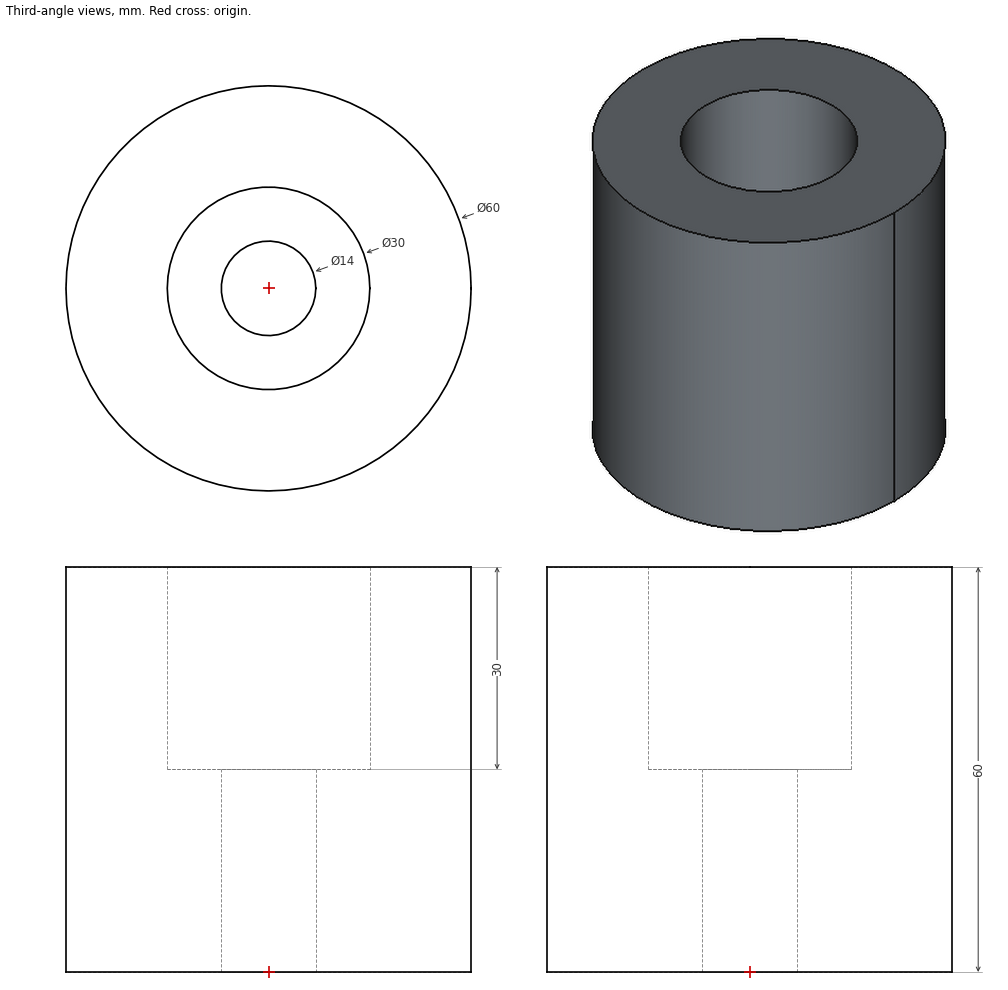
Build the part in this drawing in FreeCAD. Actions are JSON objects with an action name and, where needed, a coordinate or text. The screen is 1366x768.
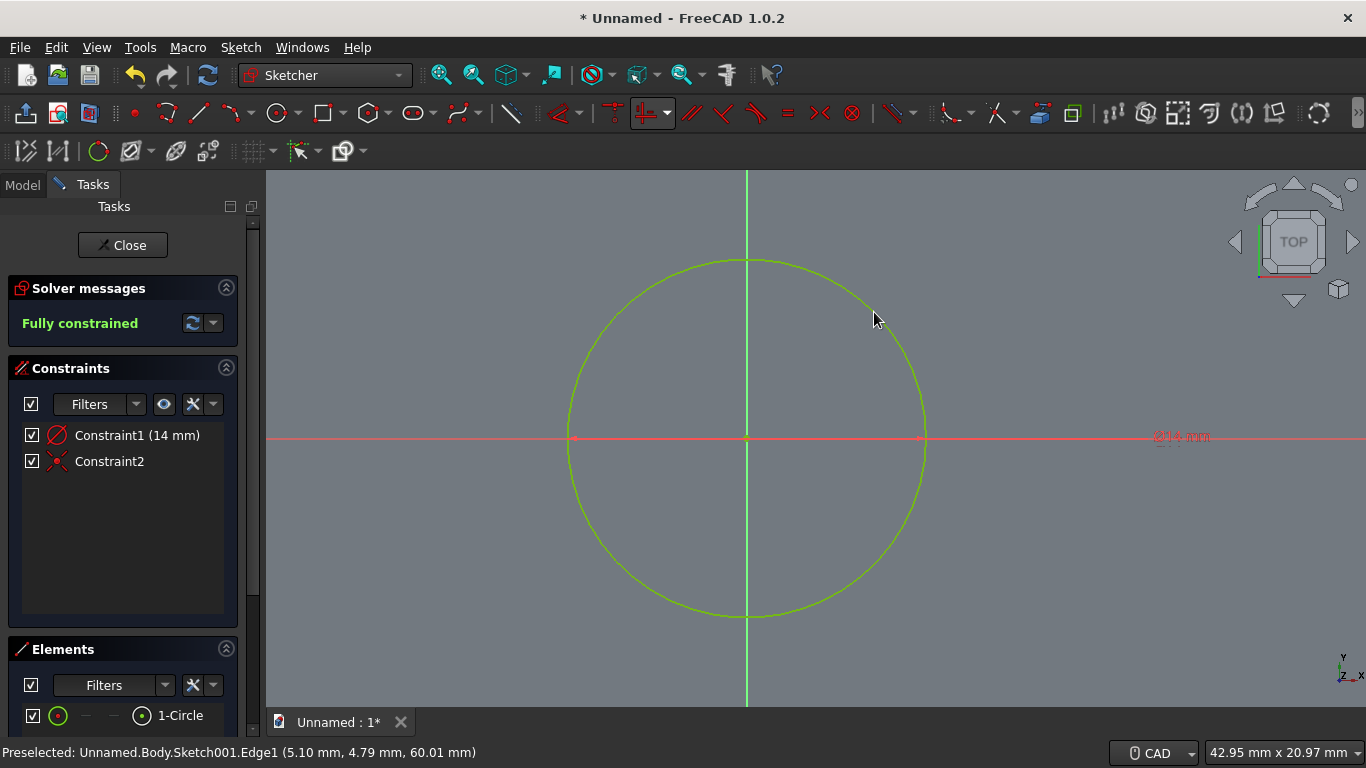
{"action": "left_click", "coordinate": [123, 245]}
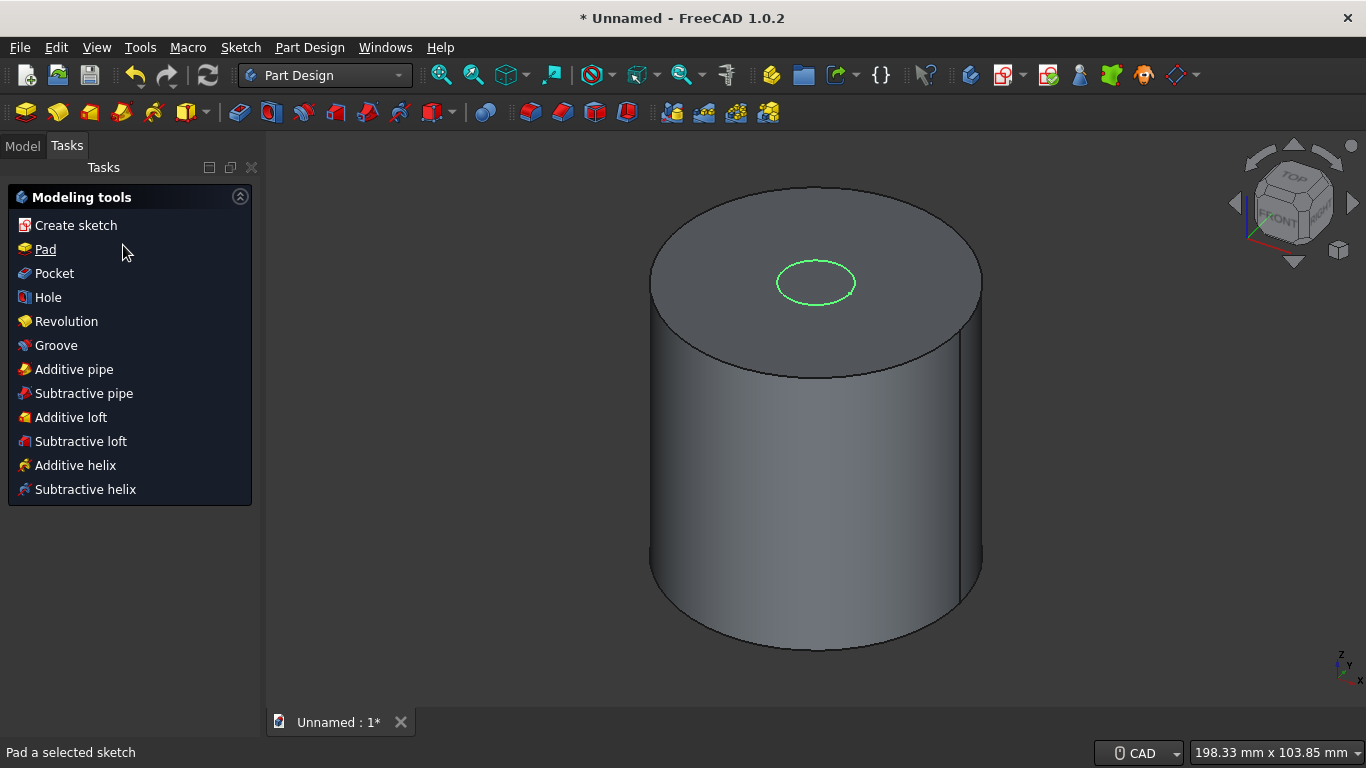
{"action": "left_click", "coordinate": [240, 112]}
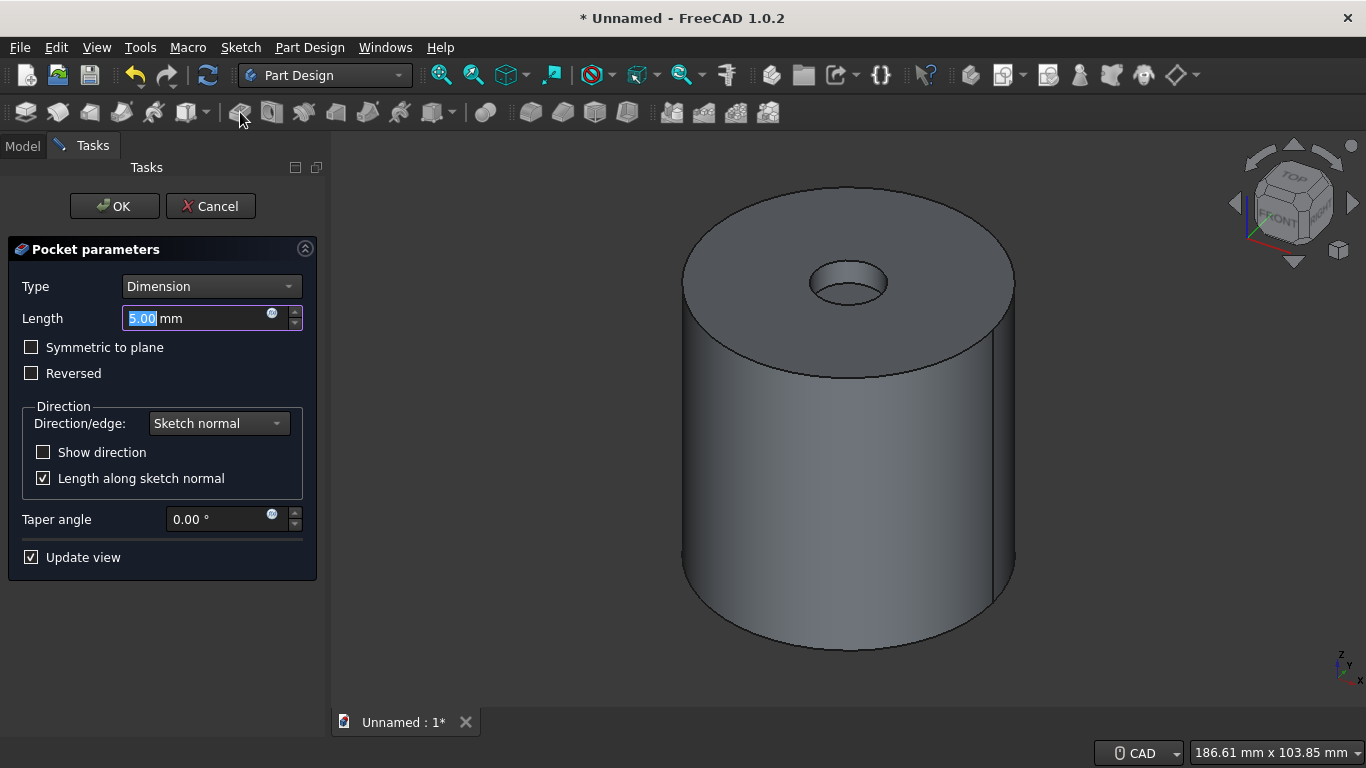
{"action": "left_click", "coordinate": [212, 286]}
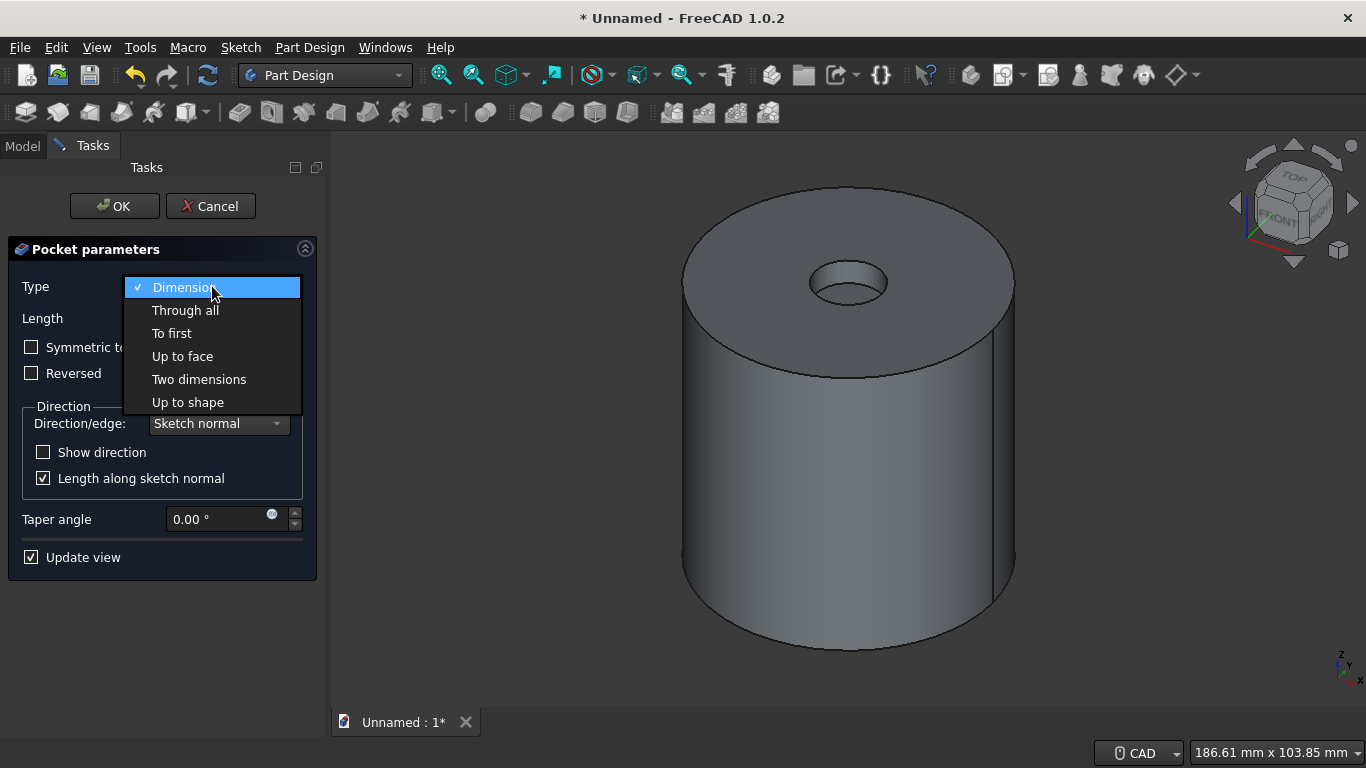
{"action": "left_click", "coordinate": [212, 310]}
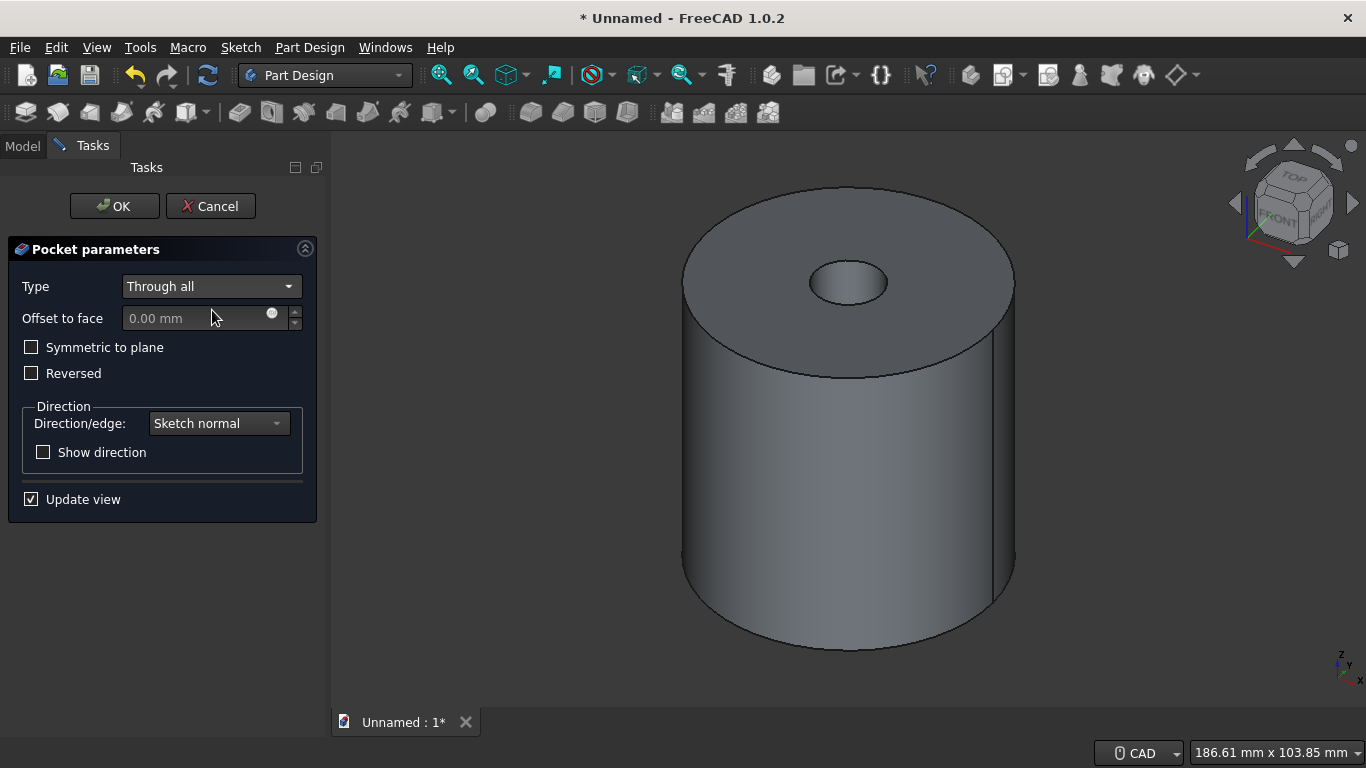
{"action": "left_click", "coordinate": [115, 206]}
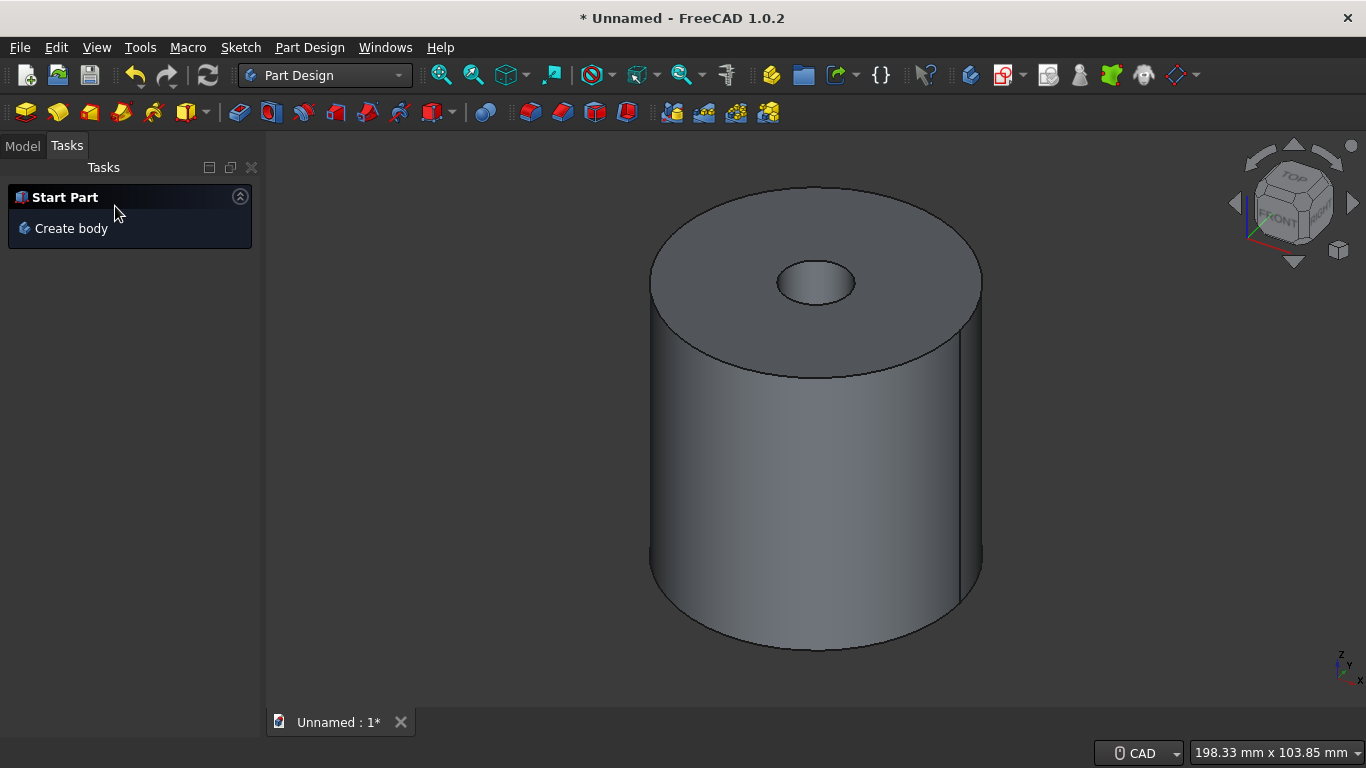
{"action": "left_click", "coordinate": [810, 343]}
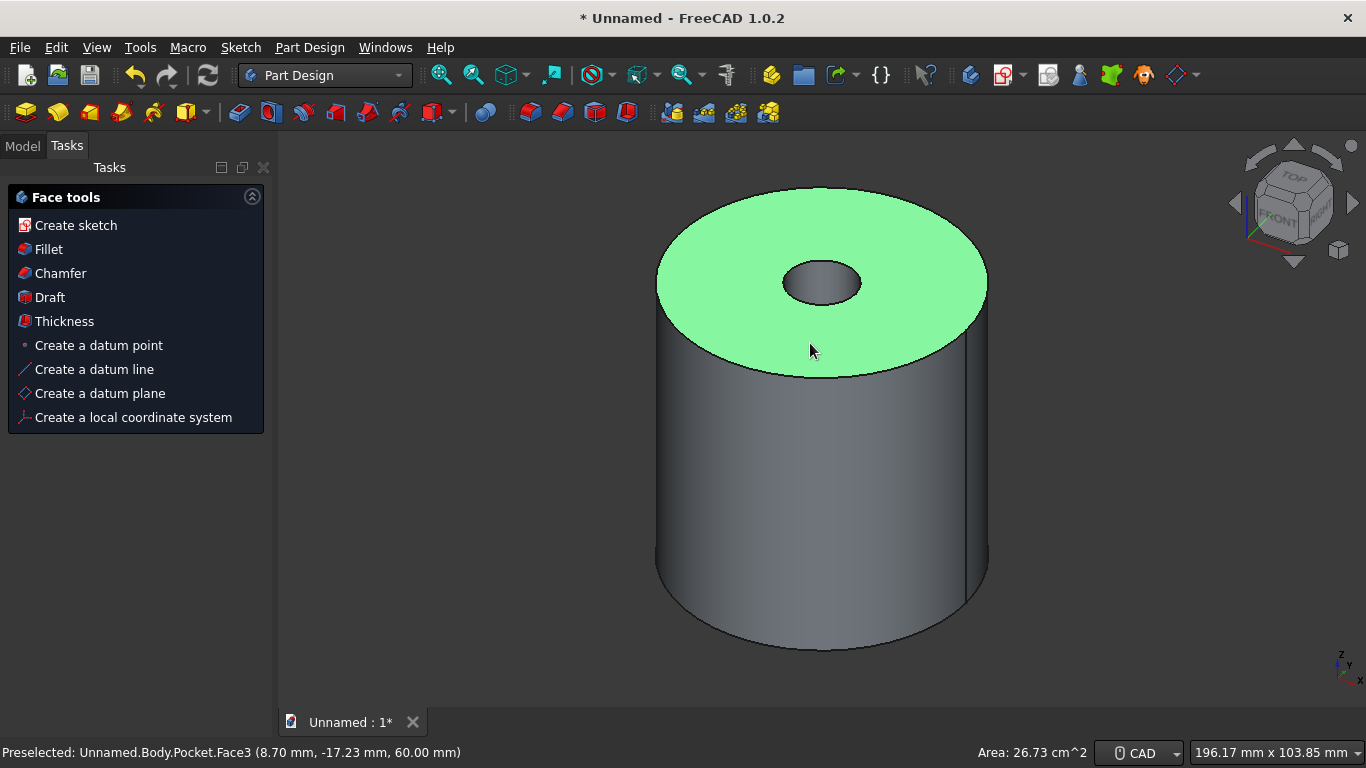
{"action": "left_click", "coordinate": [1004, 76]}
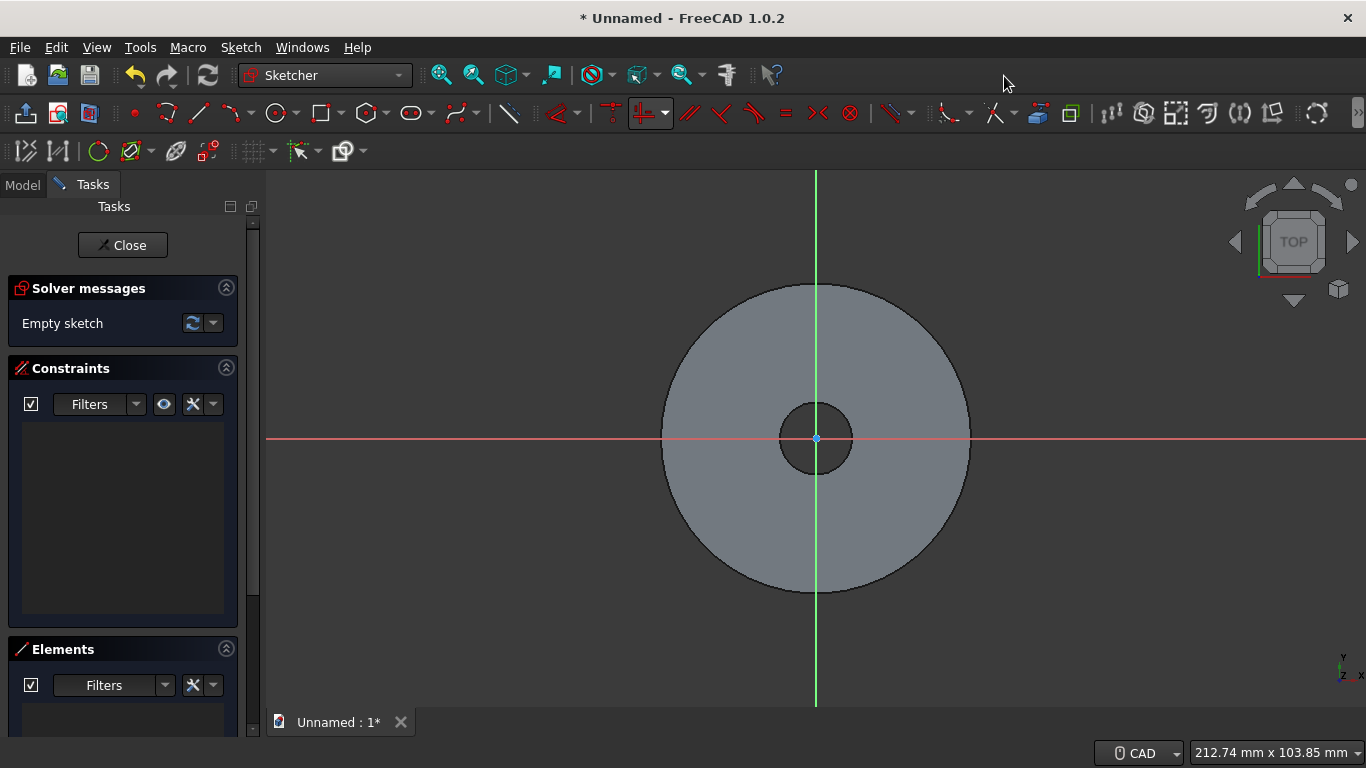
{"action": "scroll", "coordinate": [872, 438], "scroll_direction": "up", "scroll_amount": 4}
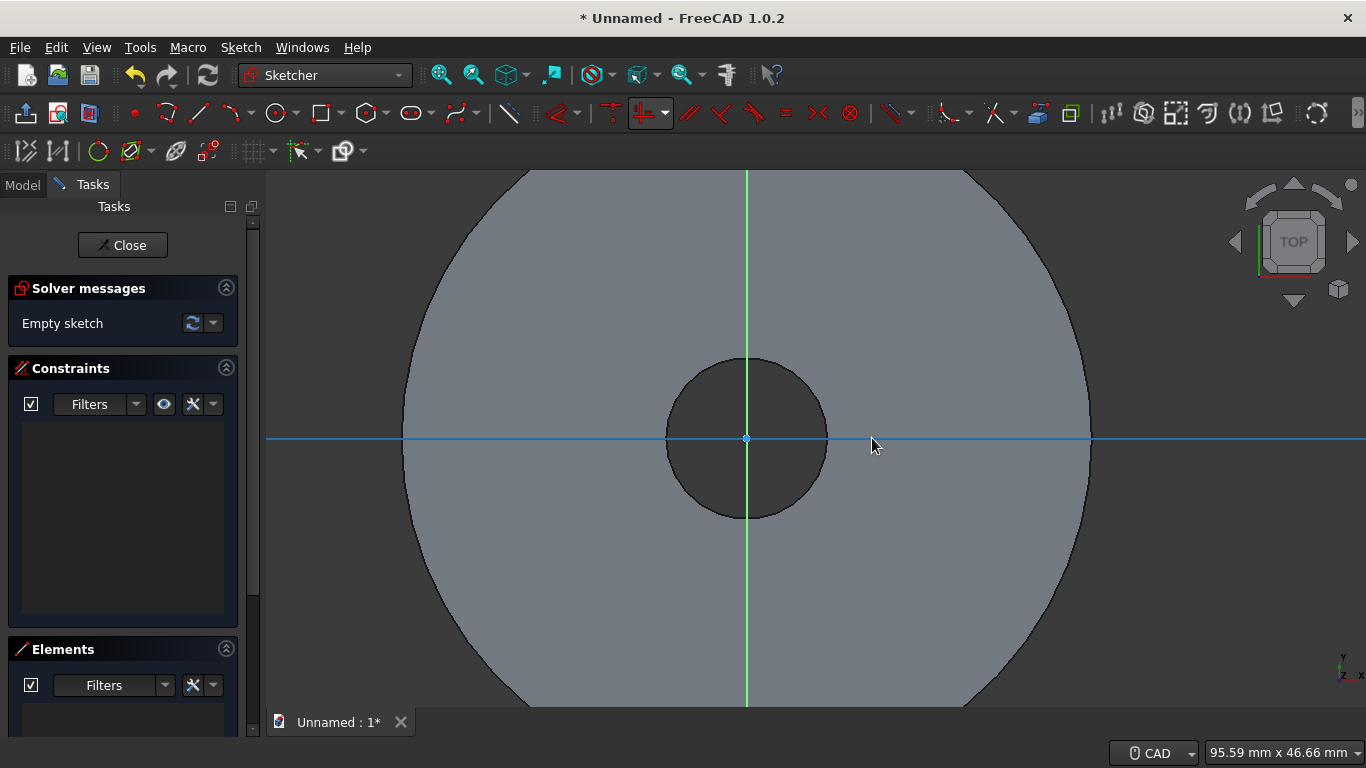
{"action": "left_click", "coordinate": [276, 114]}